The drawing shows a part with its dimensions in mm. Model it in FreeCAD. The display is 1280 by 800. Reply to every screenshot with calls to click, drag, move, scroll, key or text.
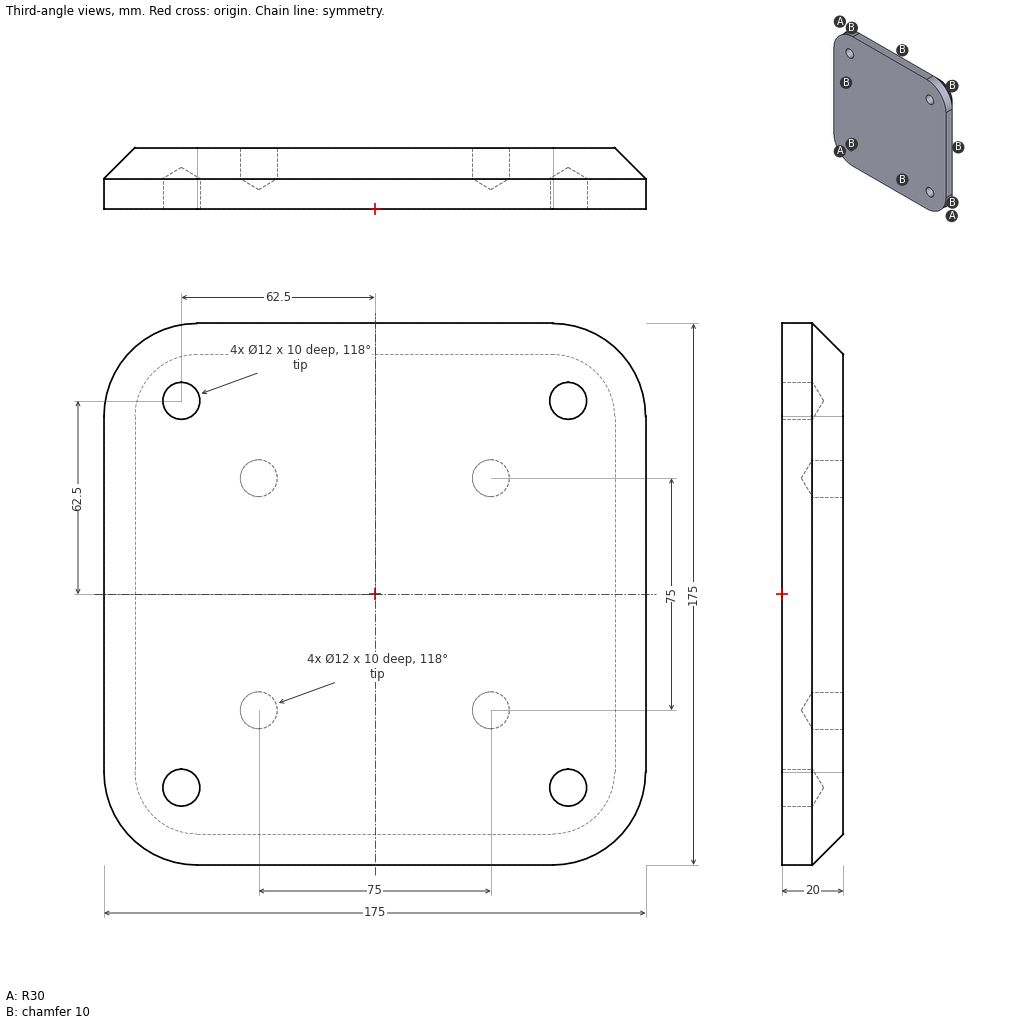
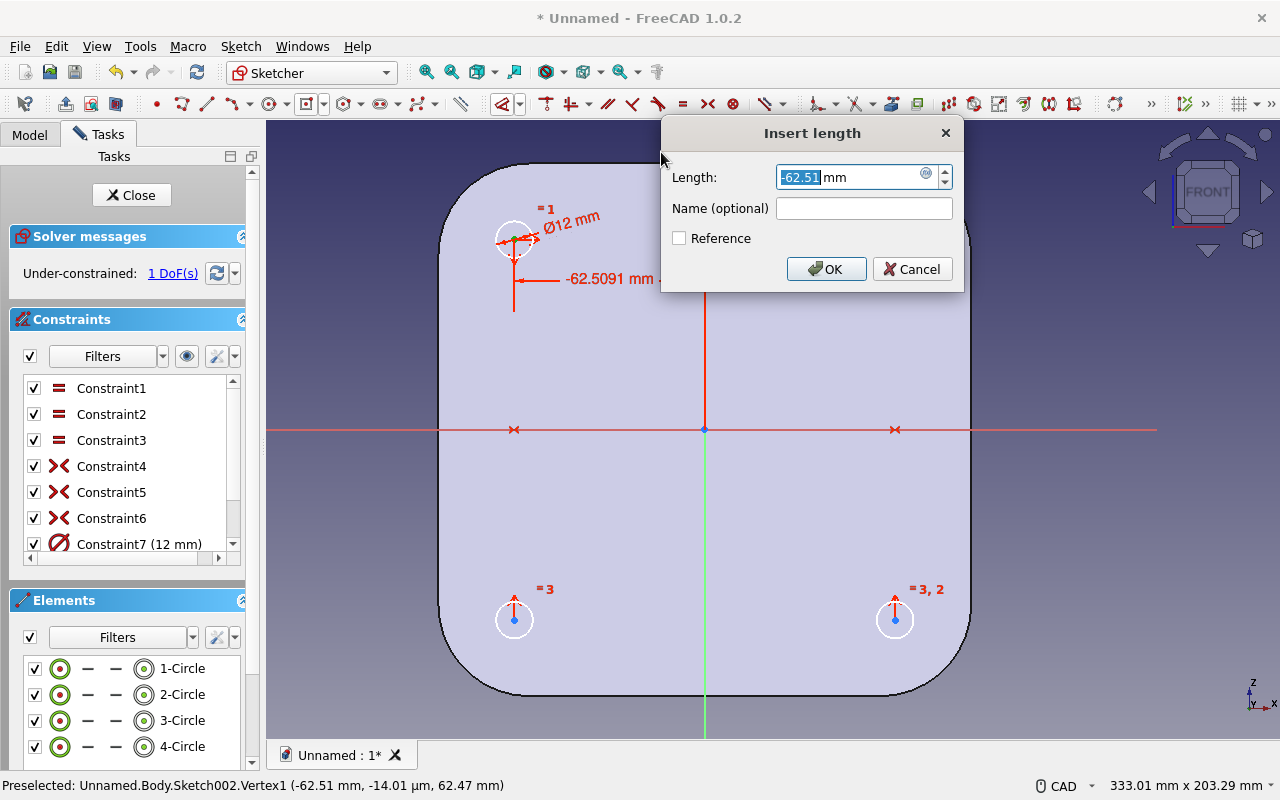
text(-62.5)
key(Return)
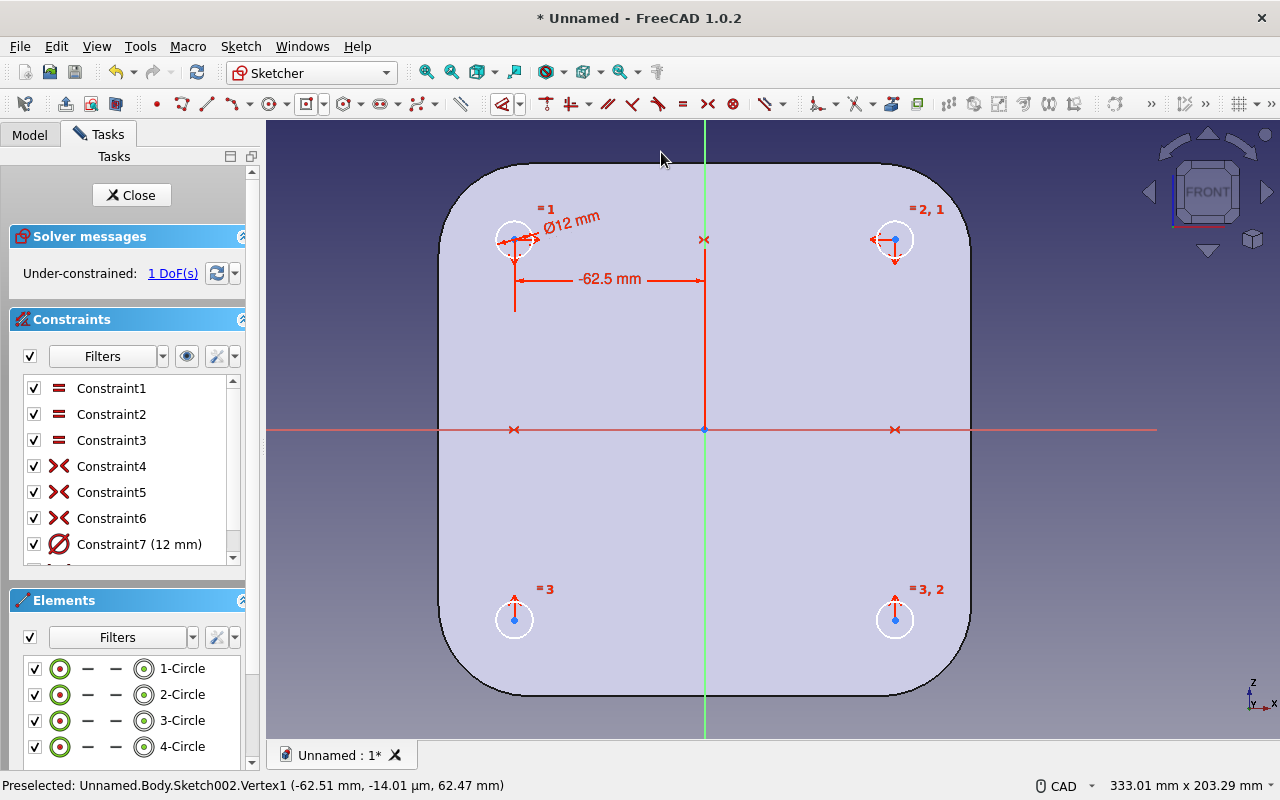
click(515, 240)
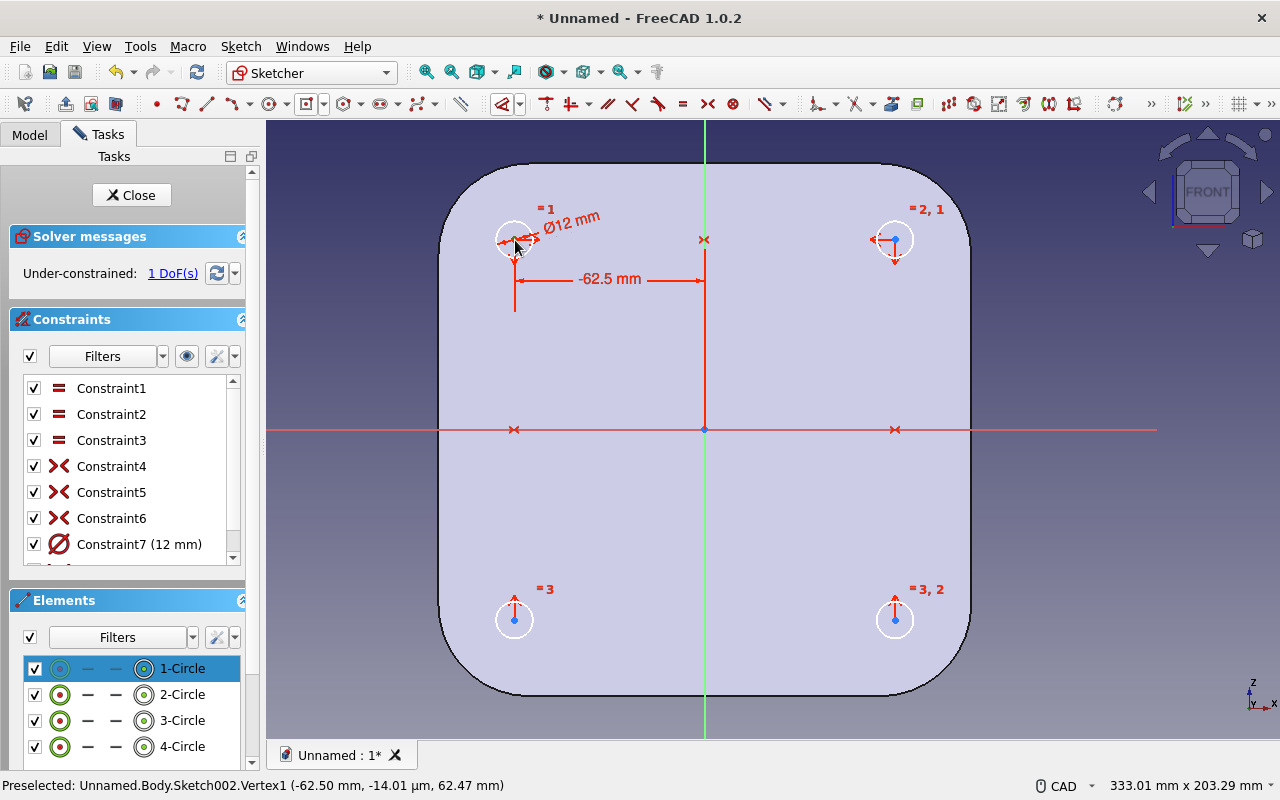
click(520, 104)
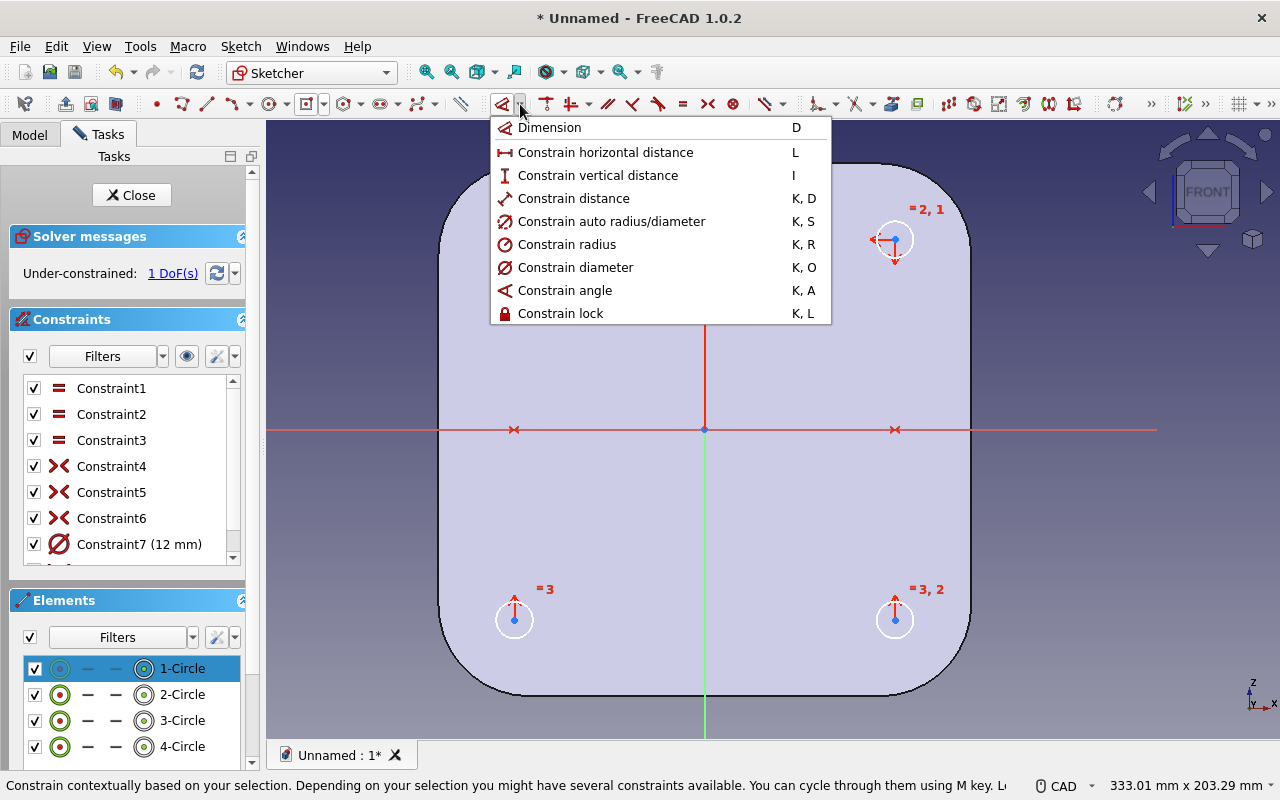
click(661, 176)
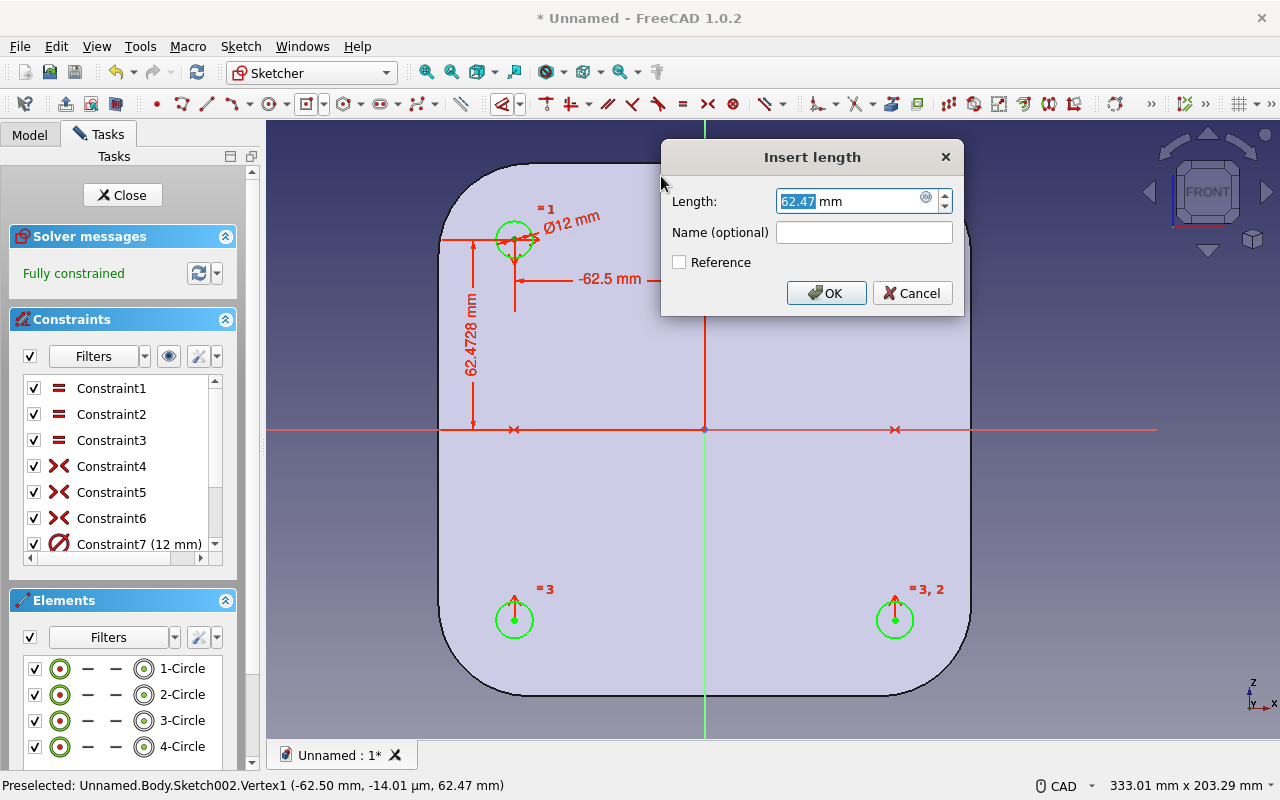
text(62.5)
key(Return)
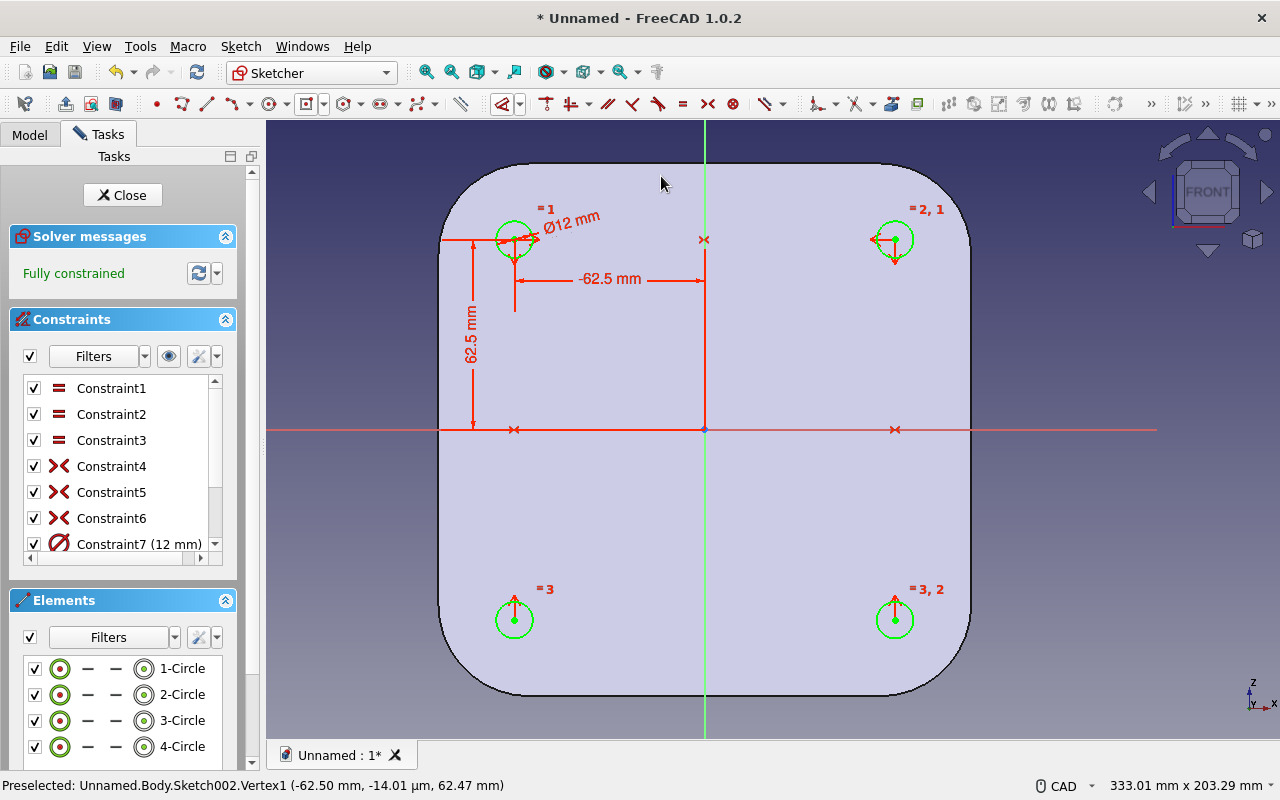
click(123, 195)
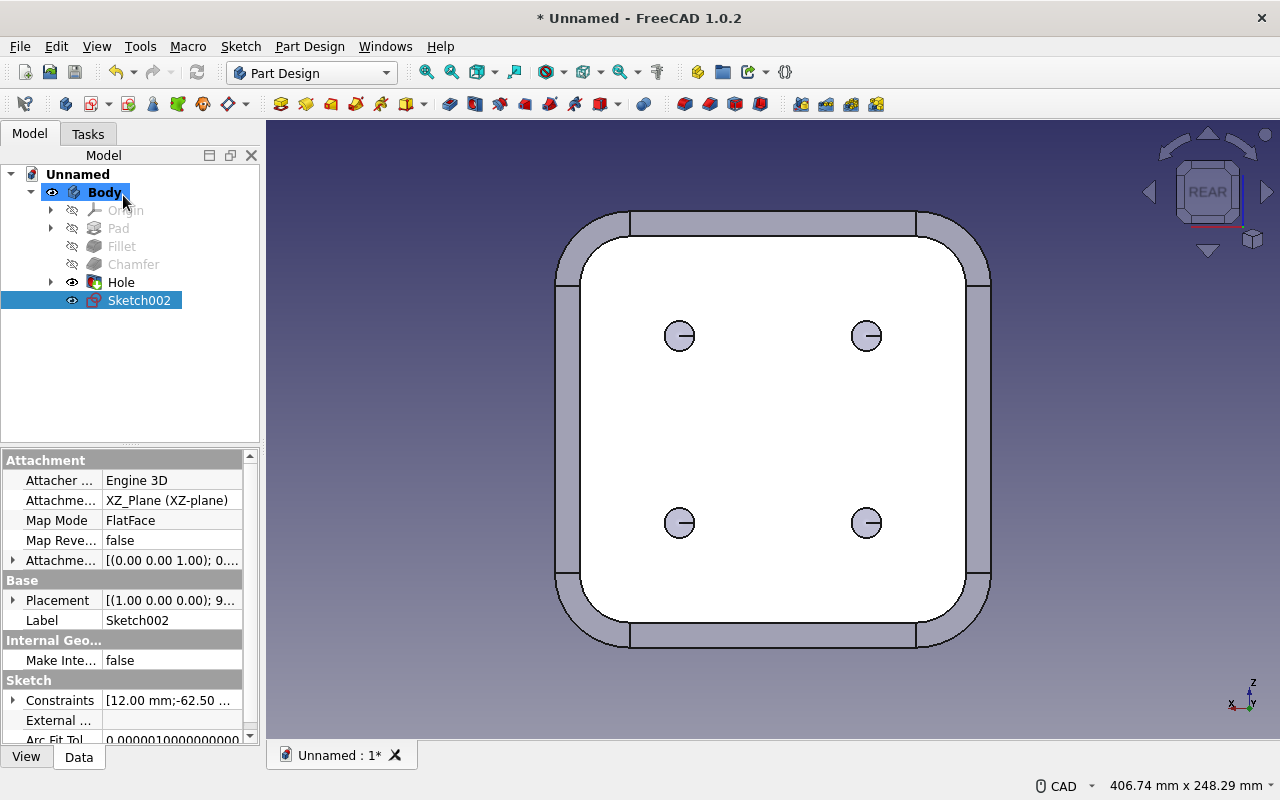
click(475, 104)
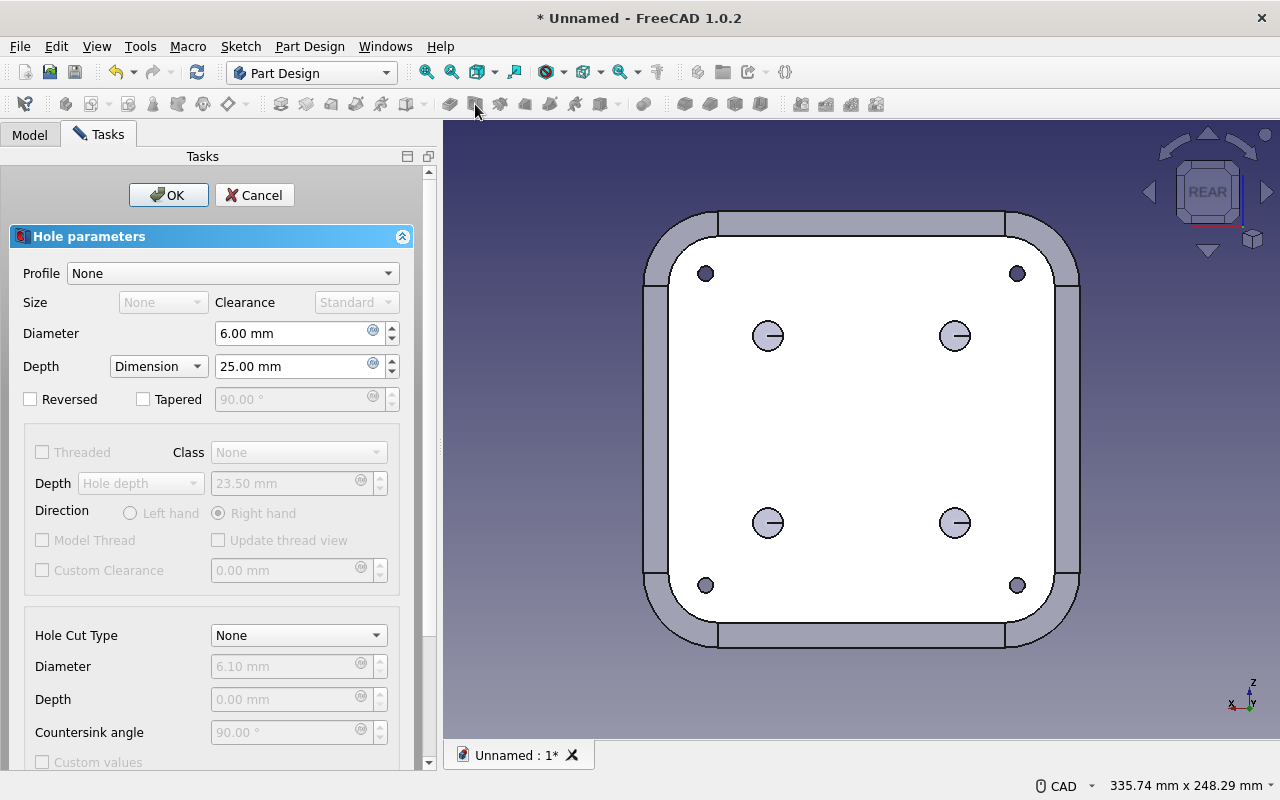
triple_click(300, 334)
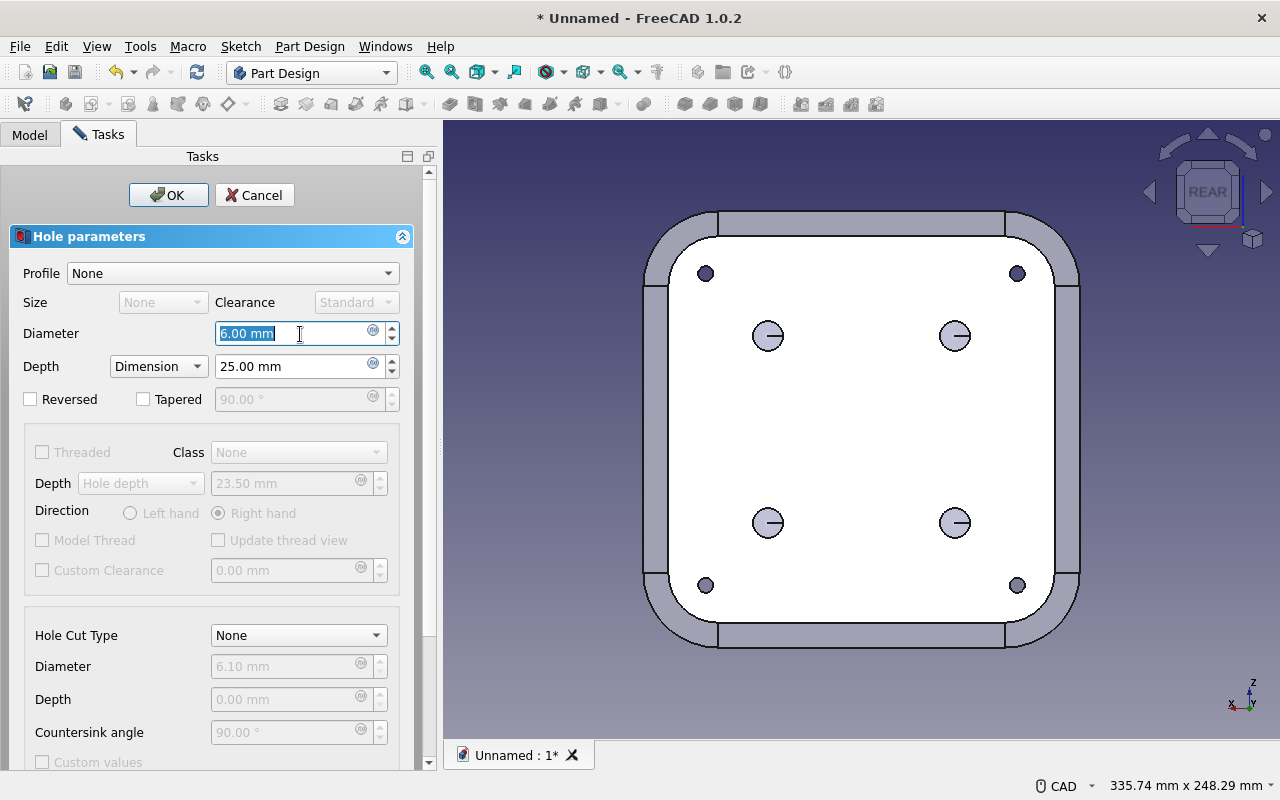
text(12)
key(Tab)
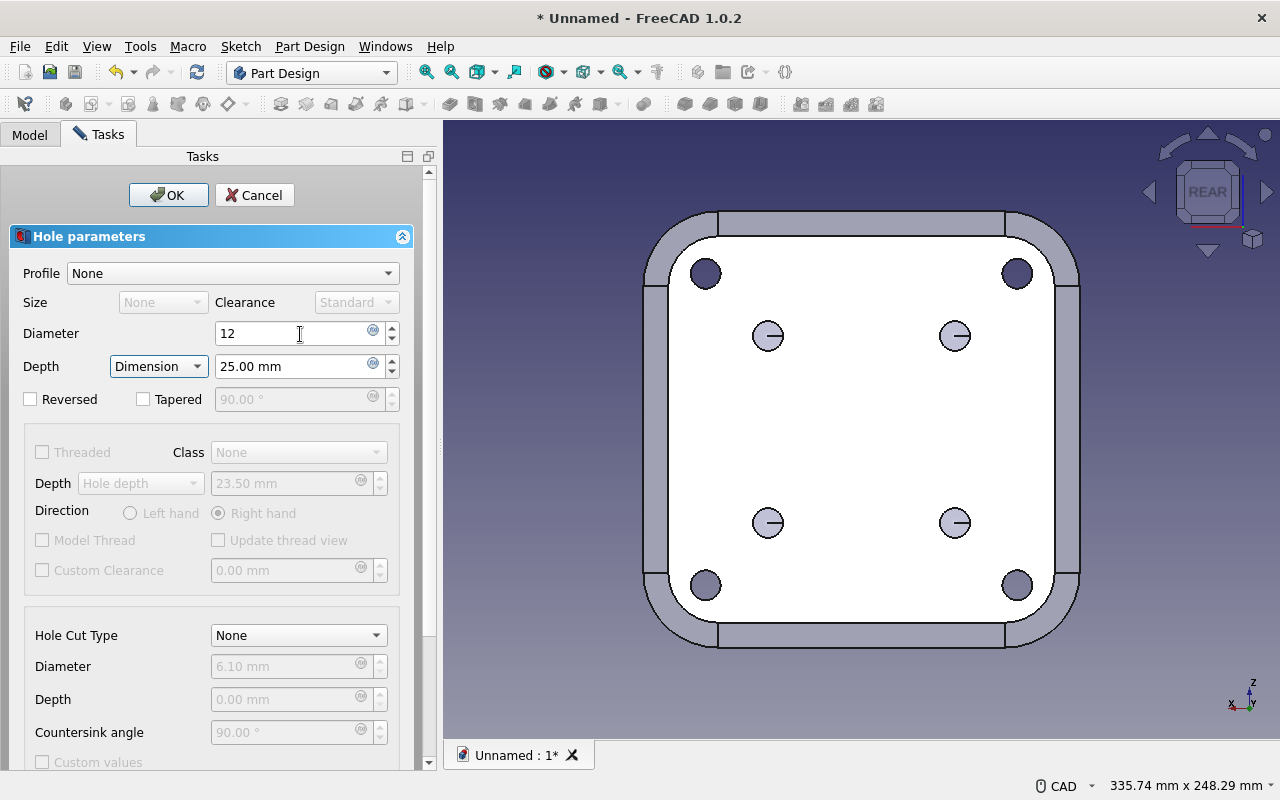
triple_click(300, 366)